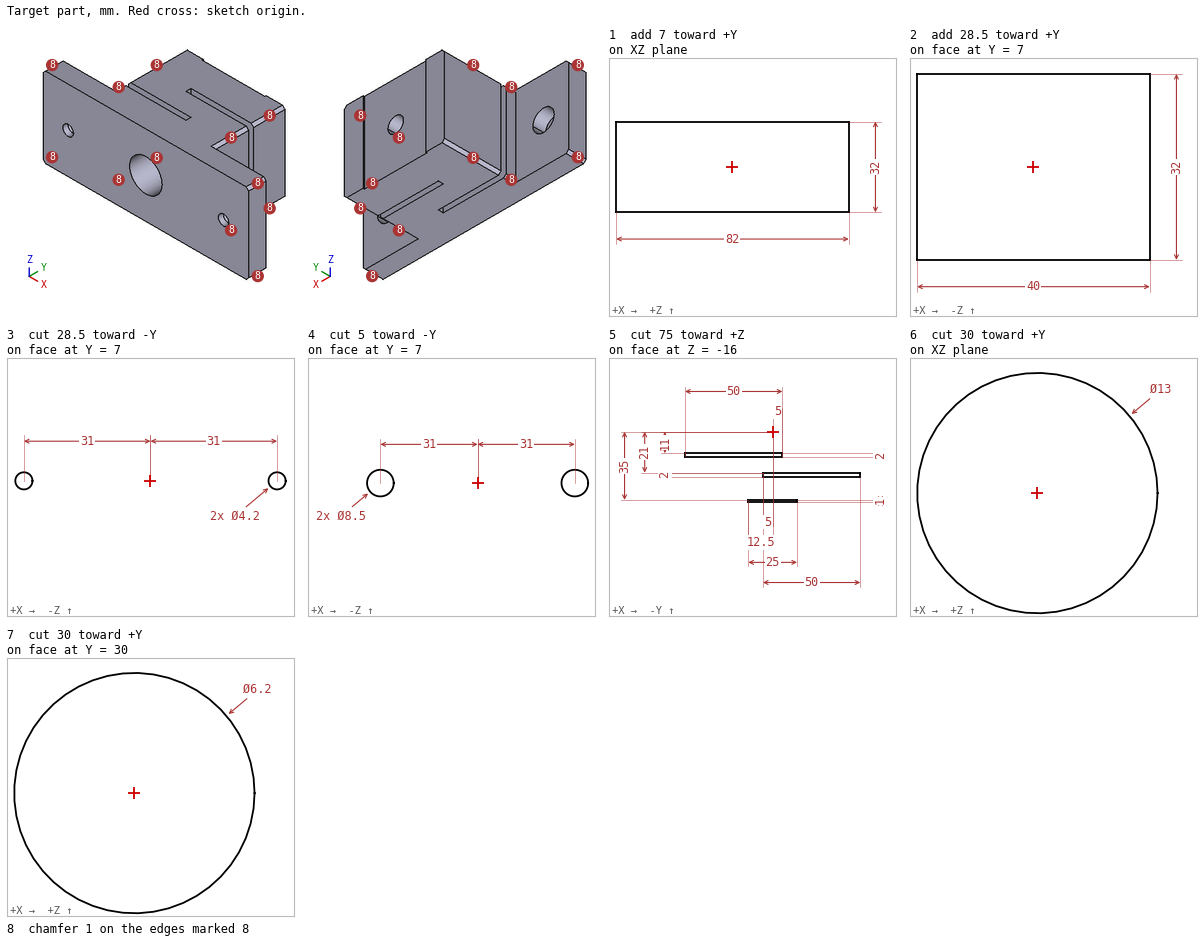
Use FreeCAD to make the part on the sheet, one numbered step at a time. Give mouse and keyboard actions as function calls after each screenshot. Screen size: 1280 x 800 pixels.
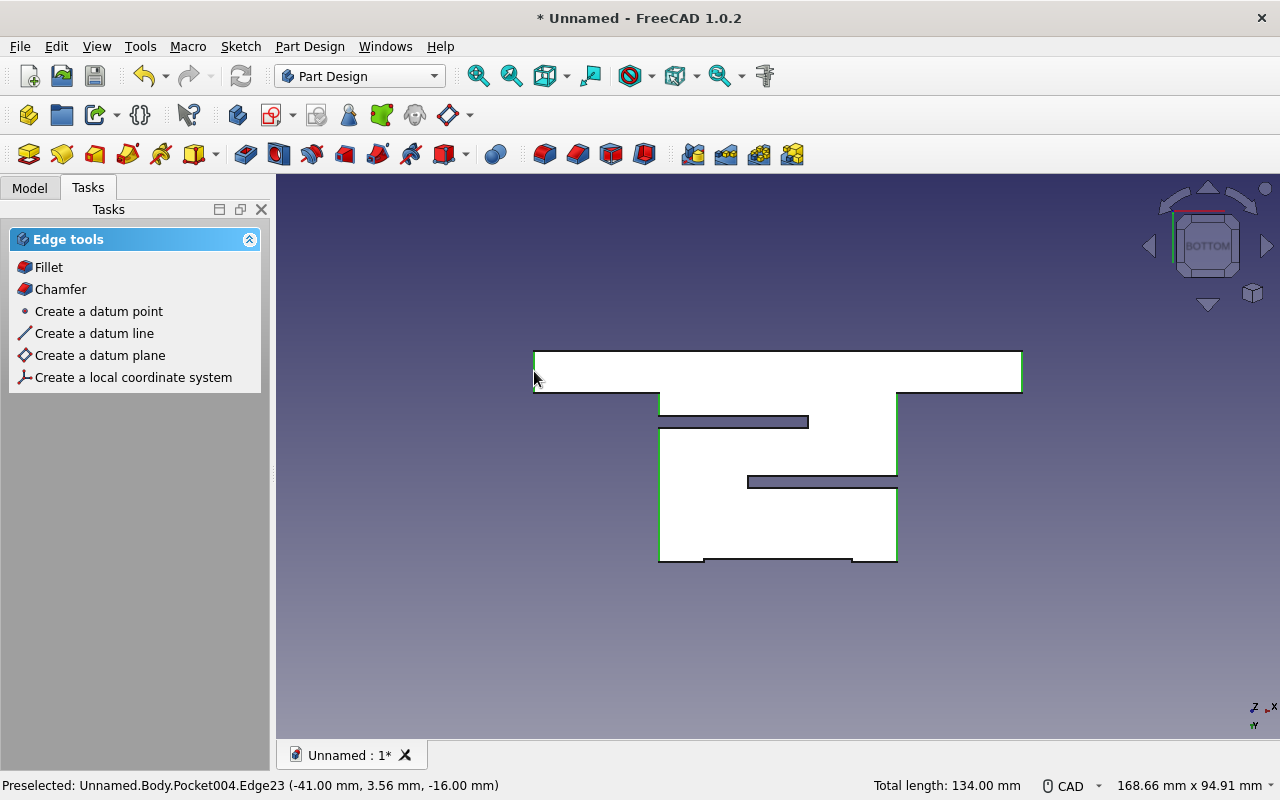
click(578, 154)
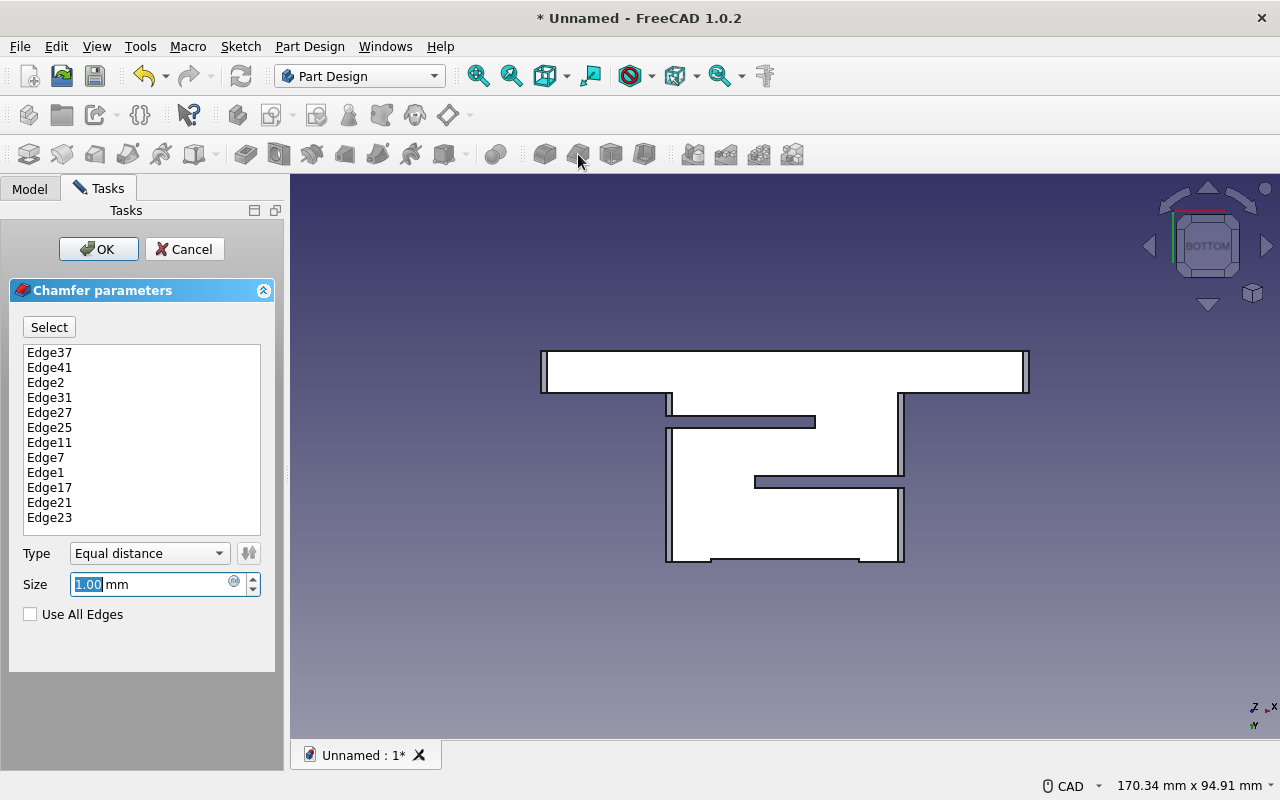
text(1)
key(Tab)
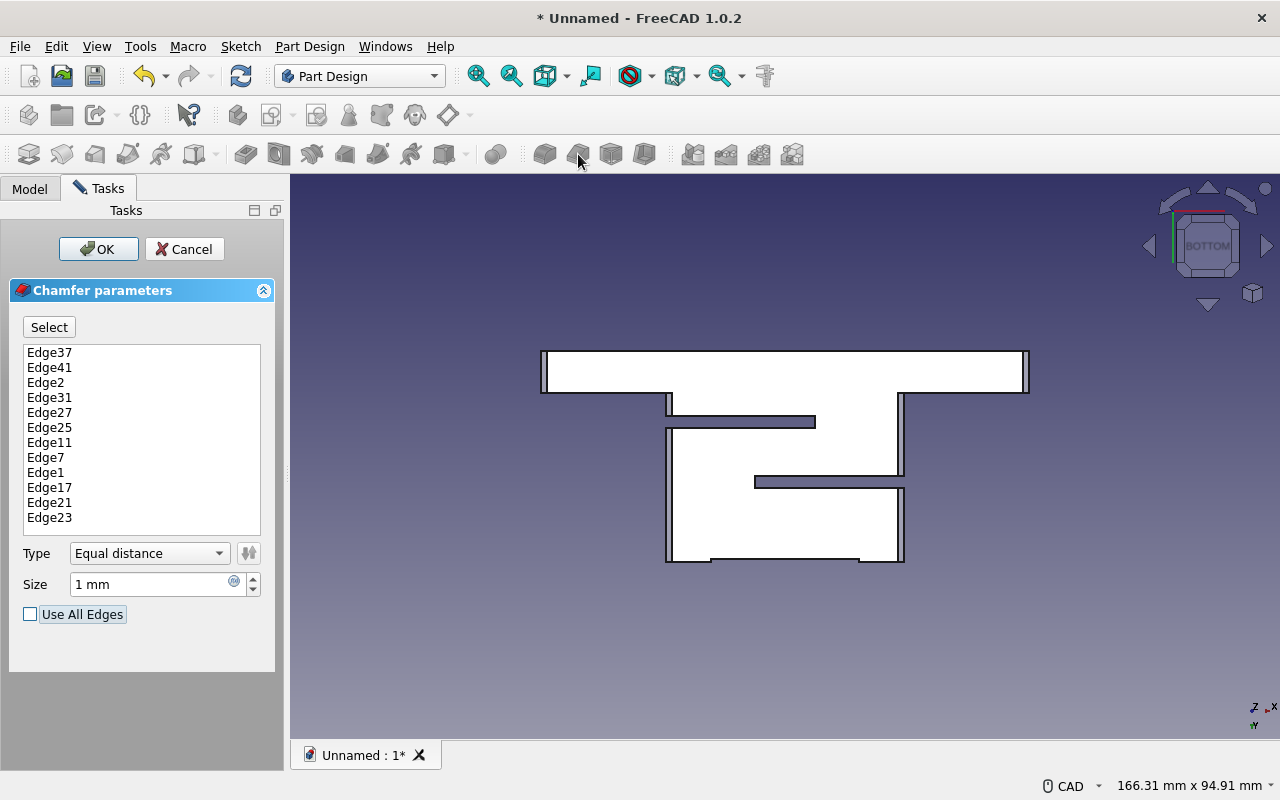
click(99, 249)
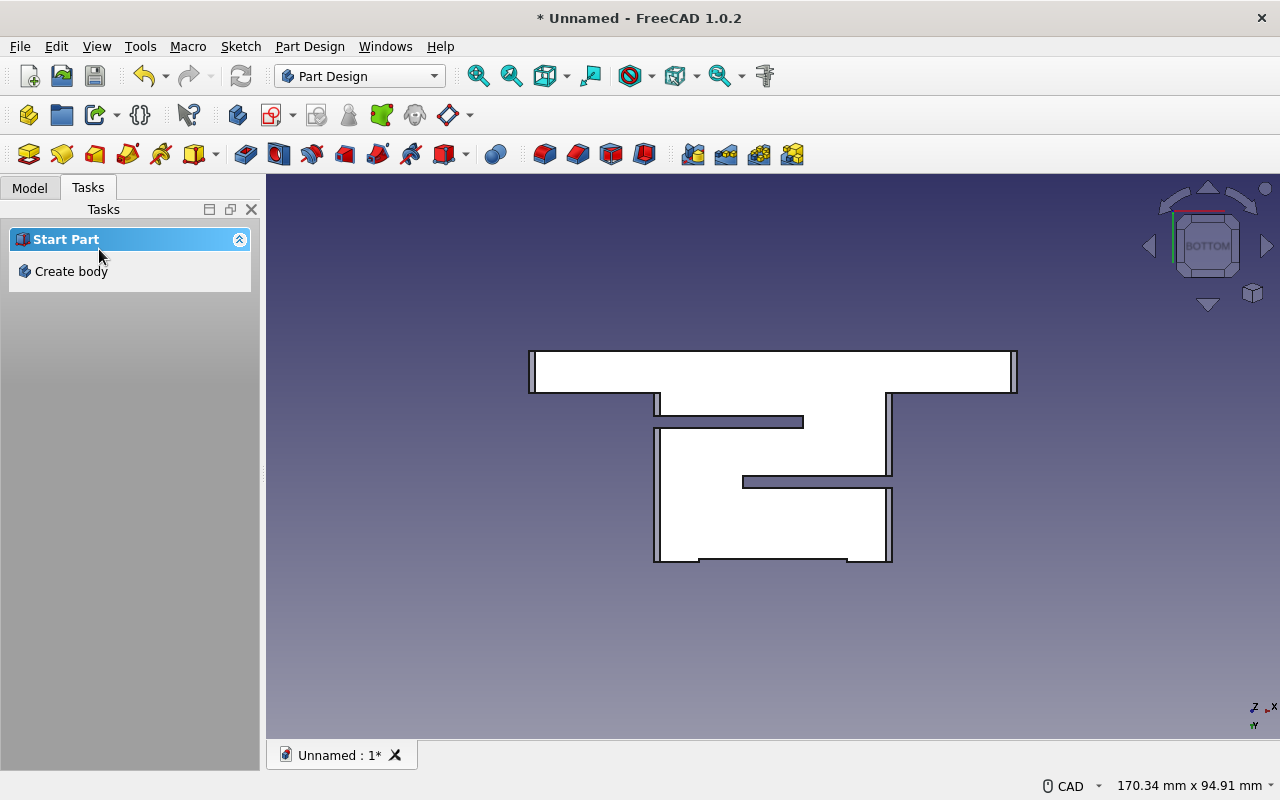
key(0)